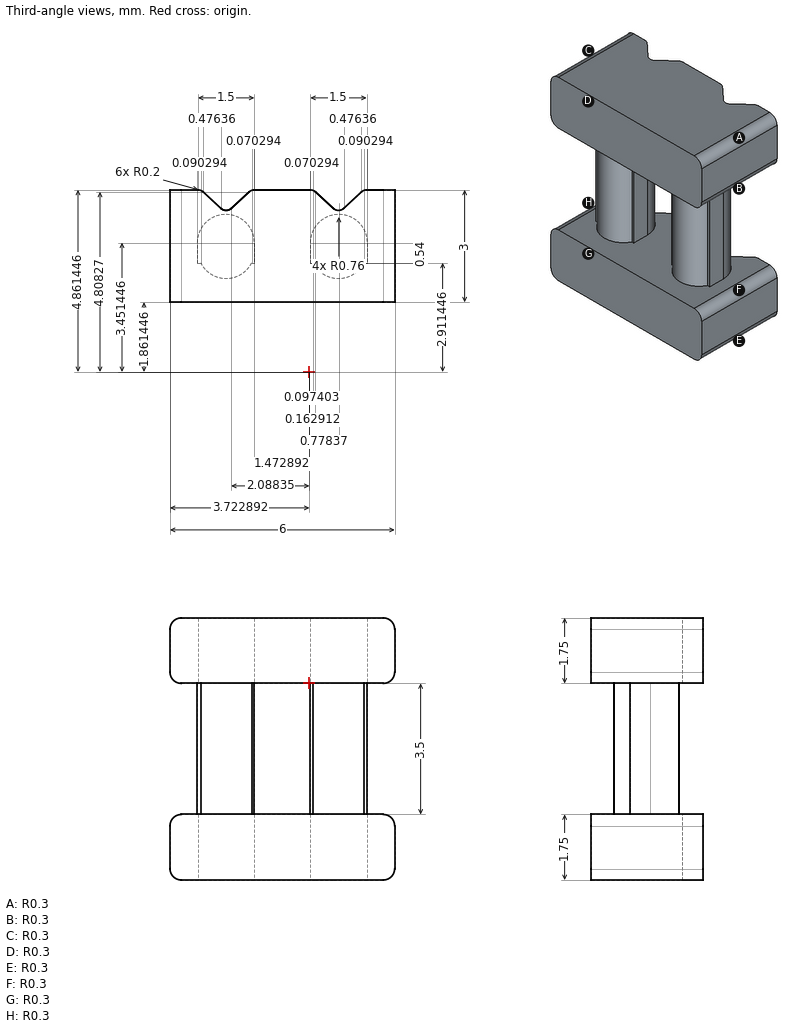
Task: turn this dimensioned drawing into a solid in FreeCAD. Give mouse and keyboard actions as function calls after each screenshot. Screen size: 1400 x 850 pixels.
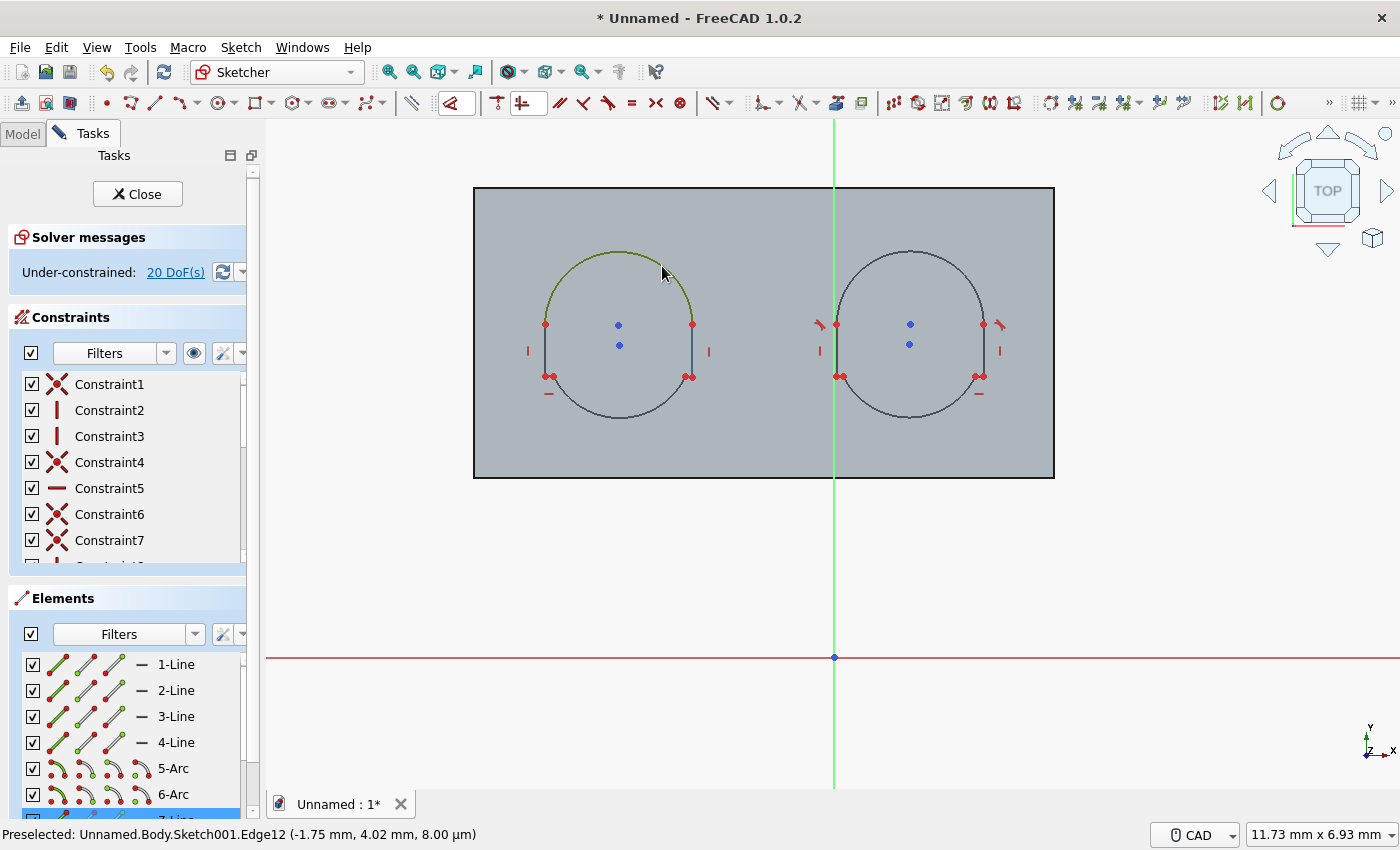
click(608, 104)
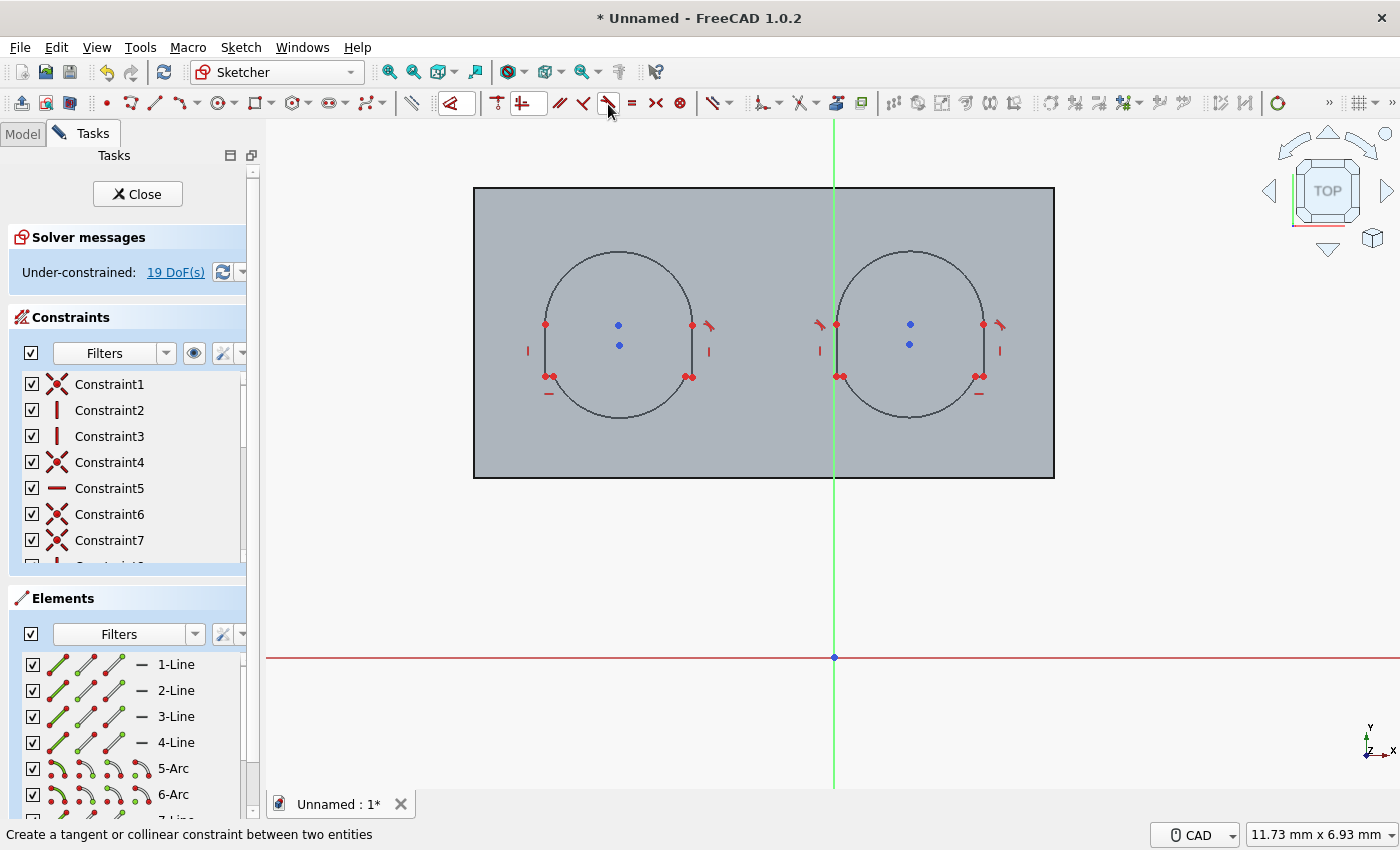
click(545, 361)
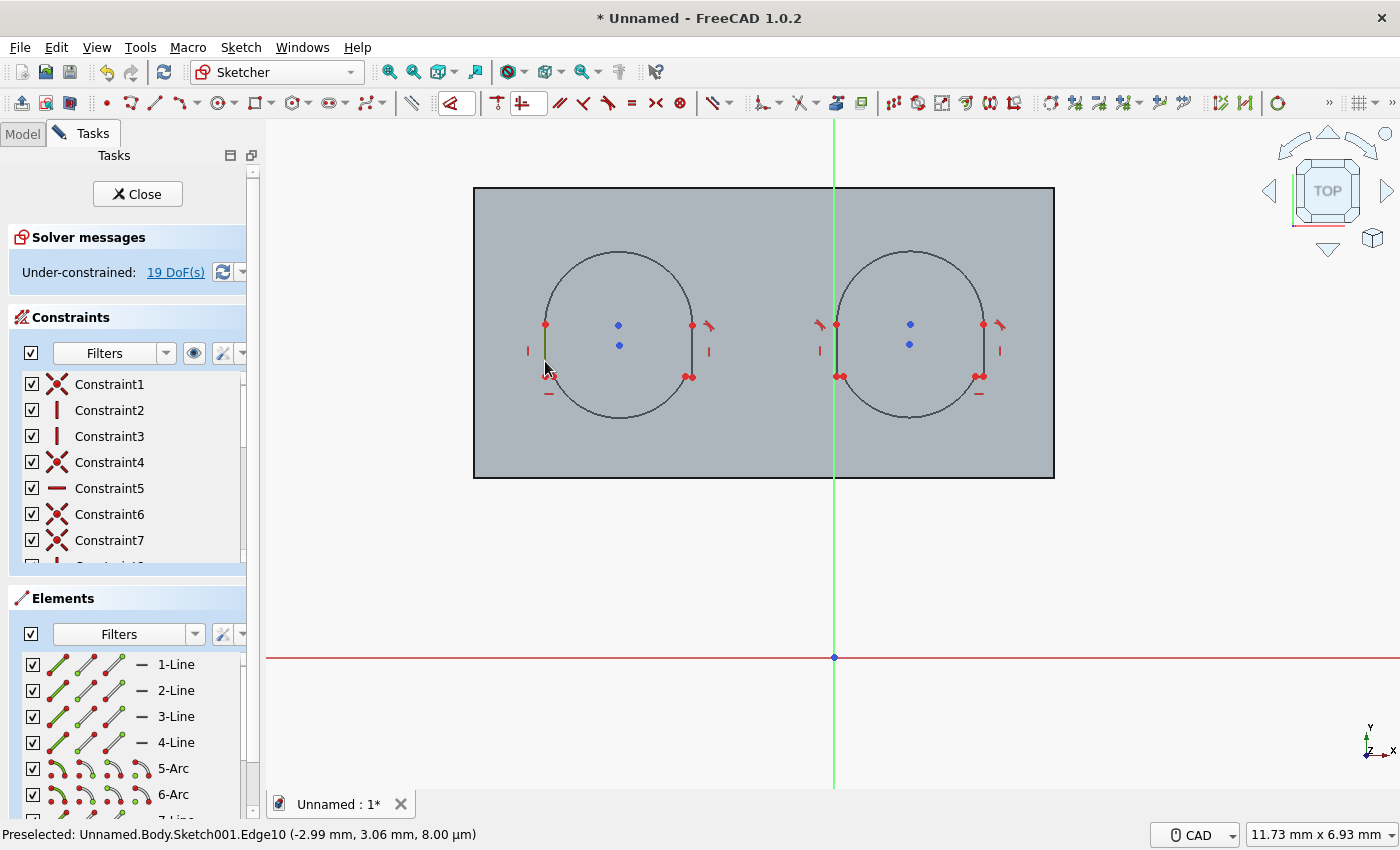
click(662, 266)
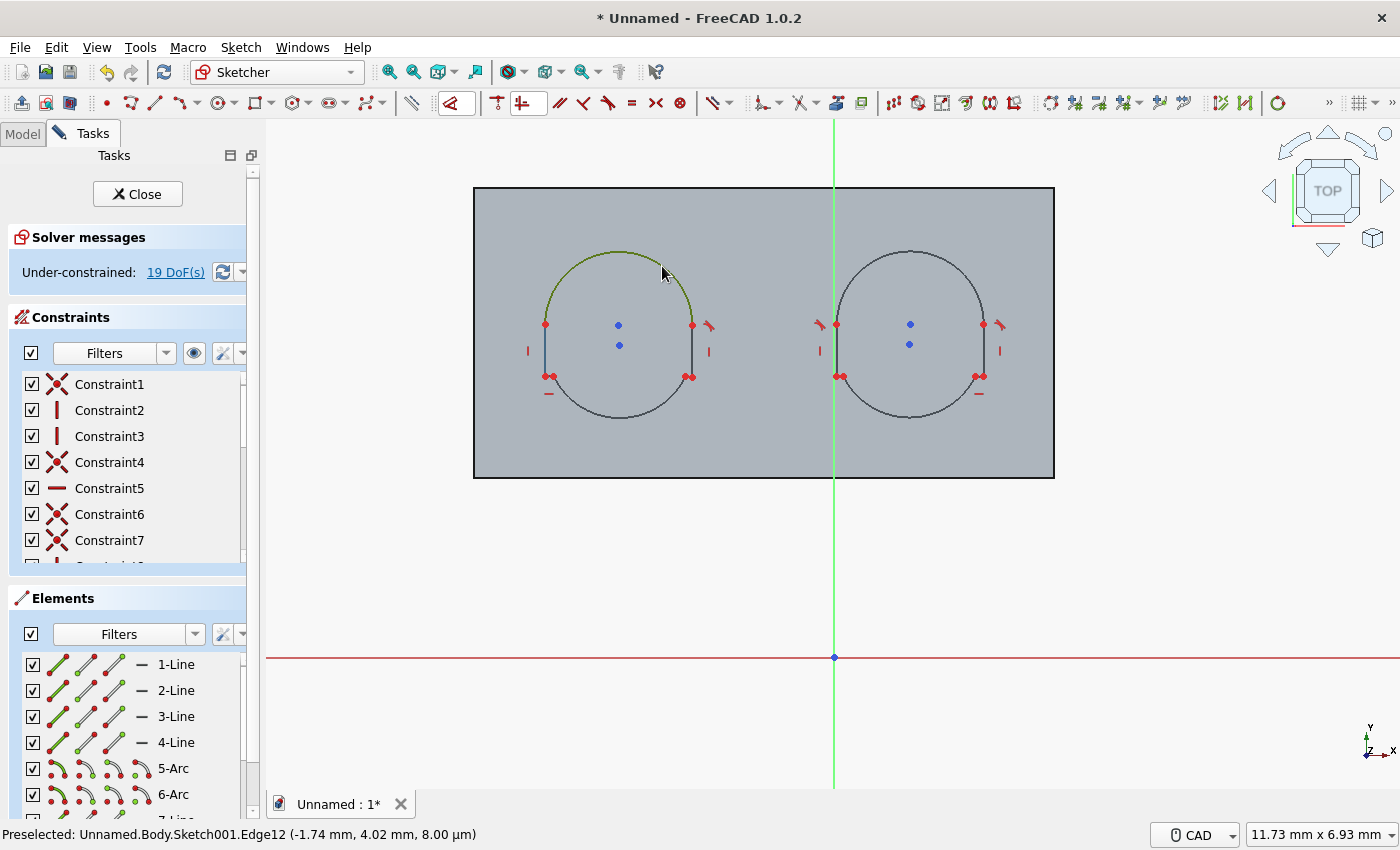
click(608, 104)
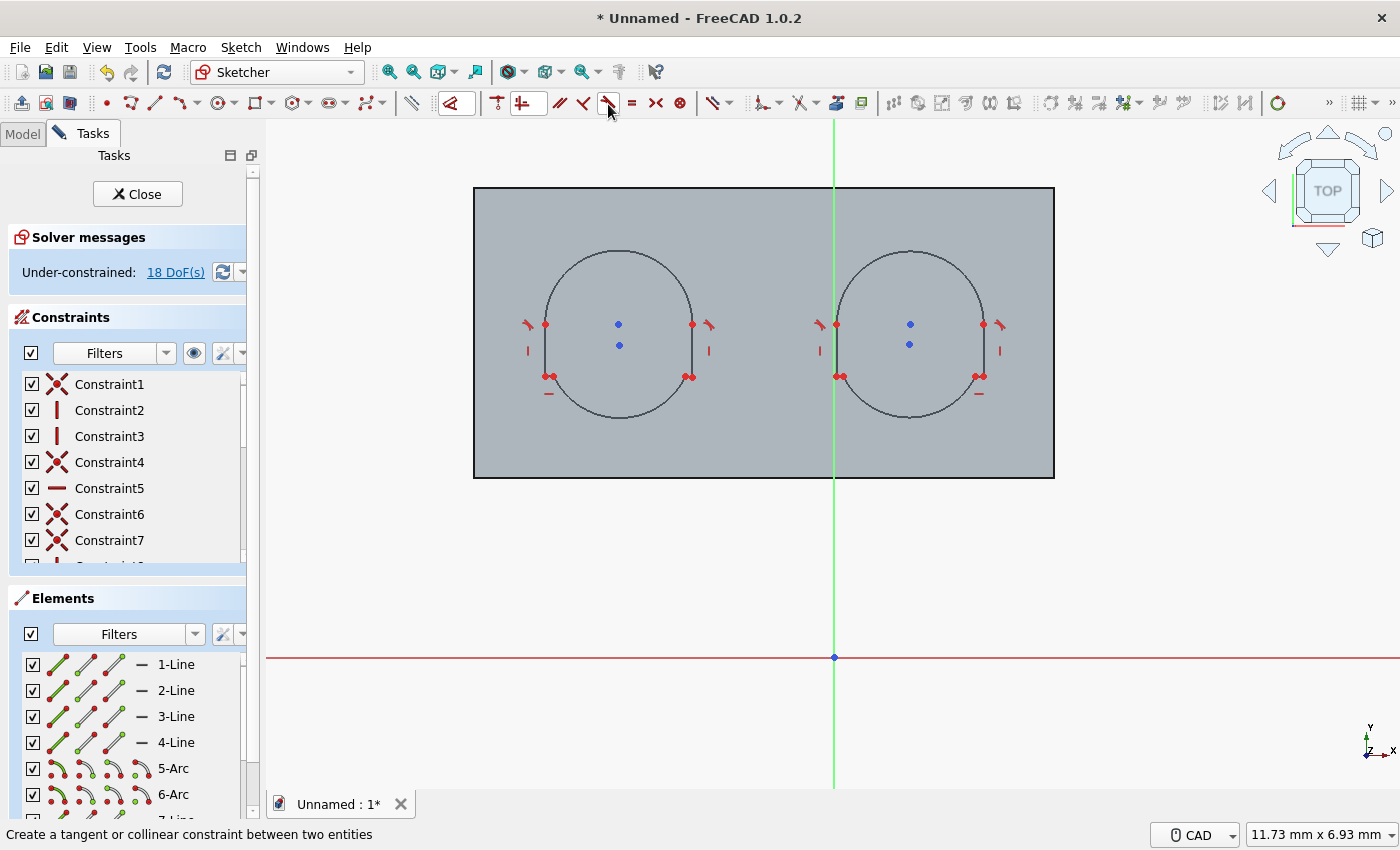
scroll(840, 376, up, 8)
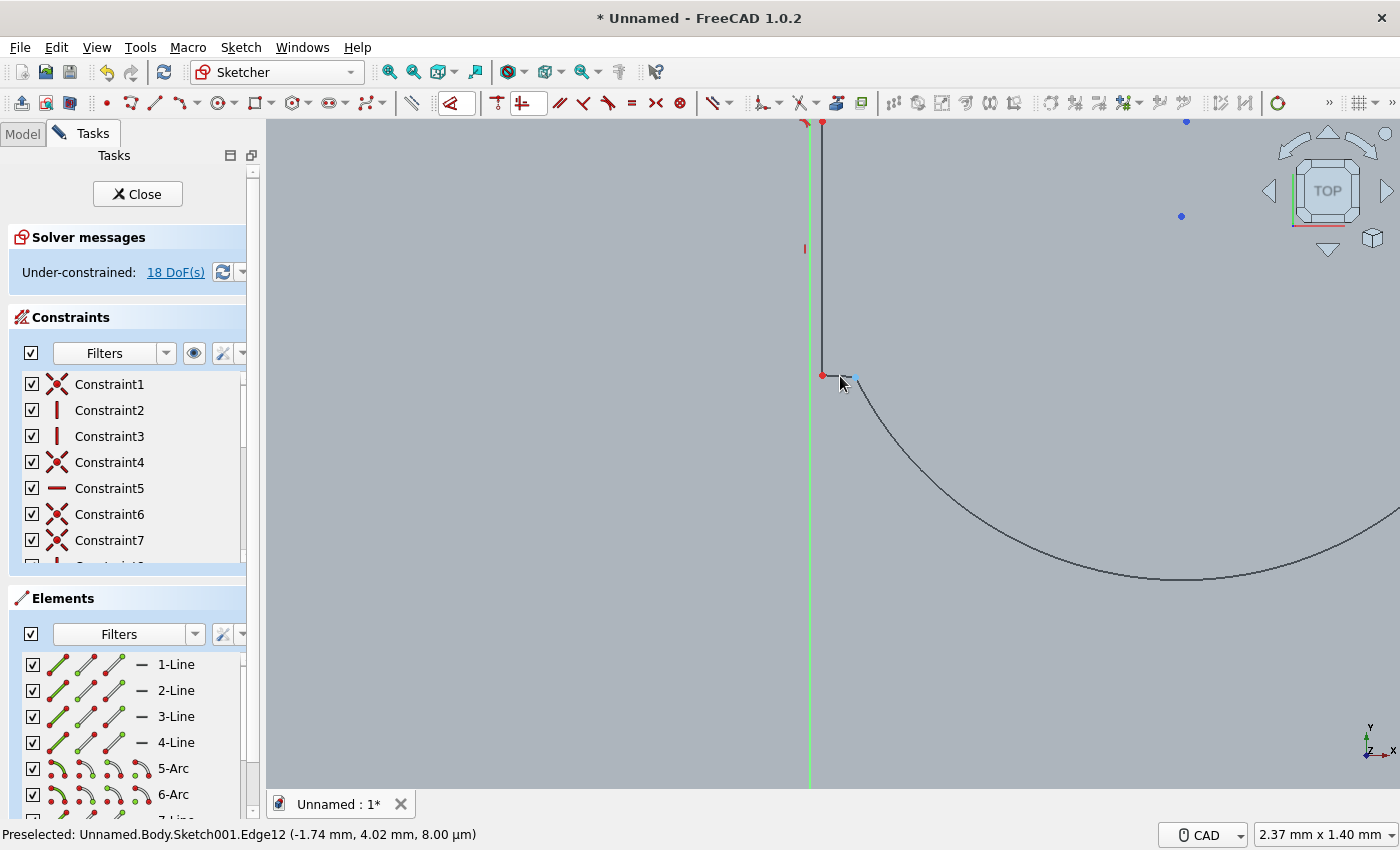
click(839, 376)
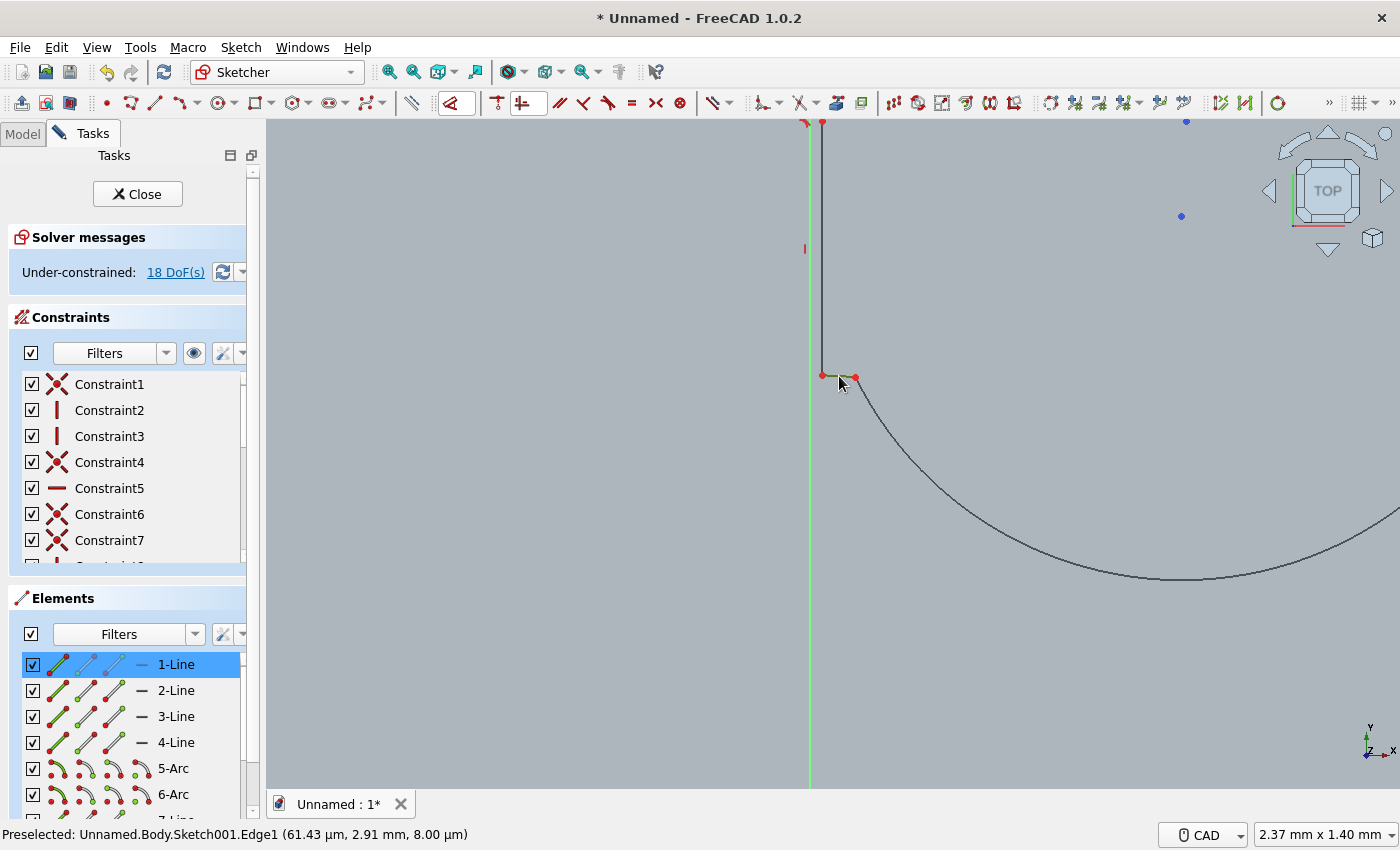
key(h)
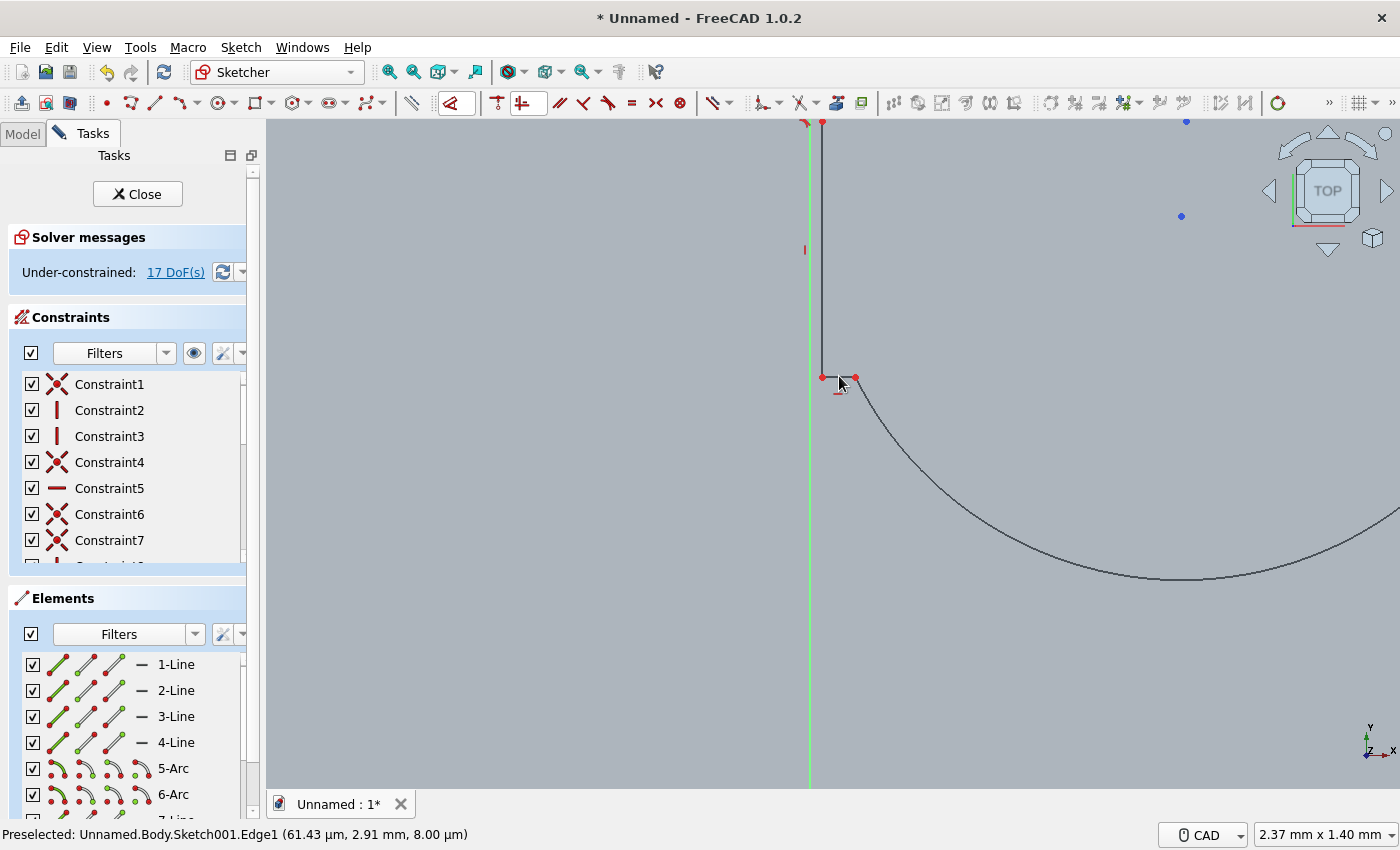
scroll(841, 376, down, 8)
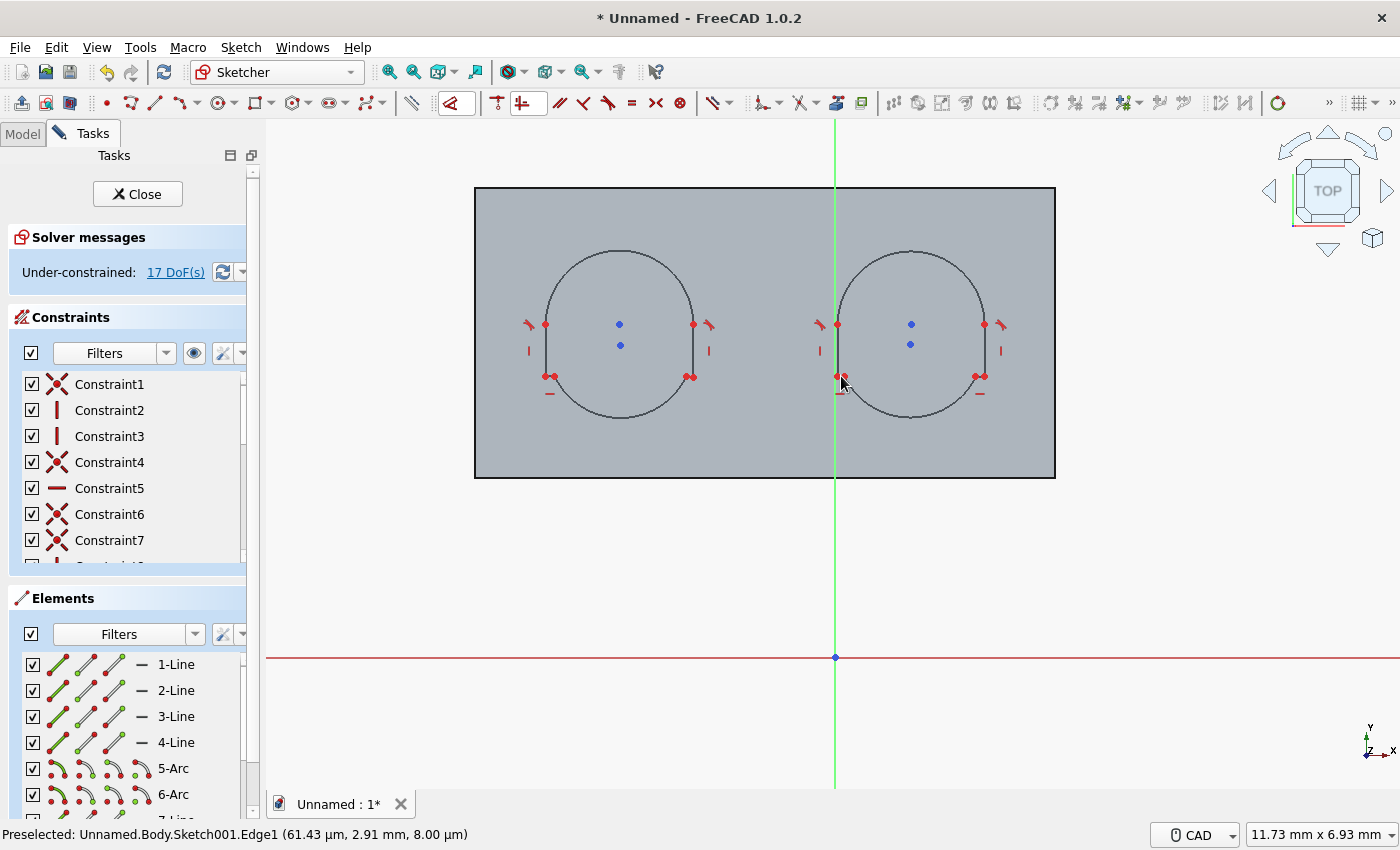
scroll(691, 377, up, 10)